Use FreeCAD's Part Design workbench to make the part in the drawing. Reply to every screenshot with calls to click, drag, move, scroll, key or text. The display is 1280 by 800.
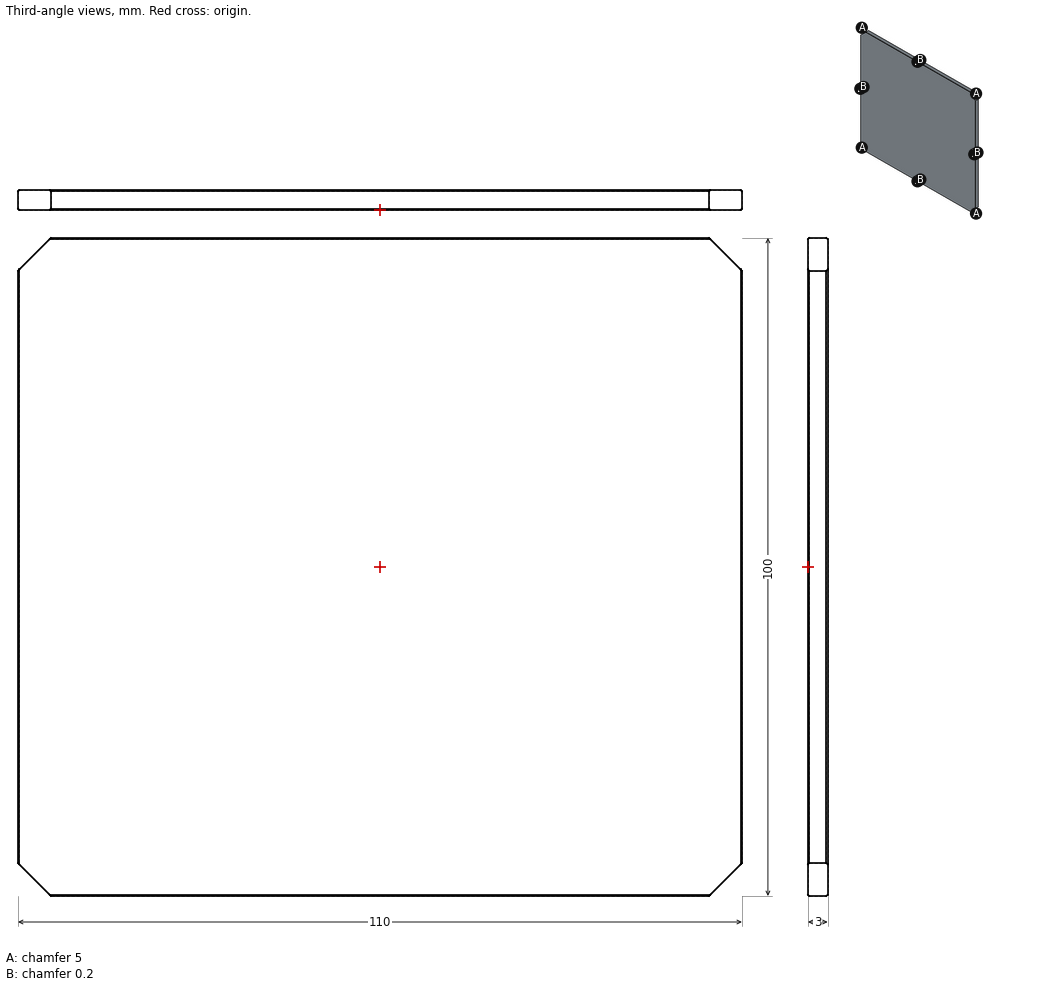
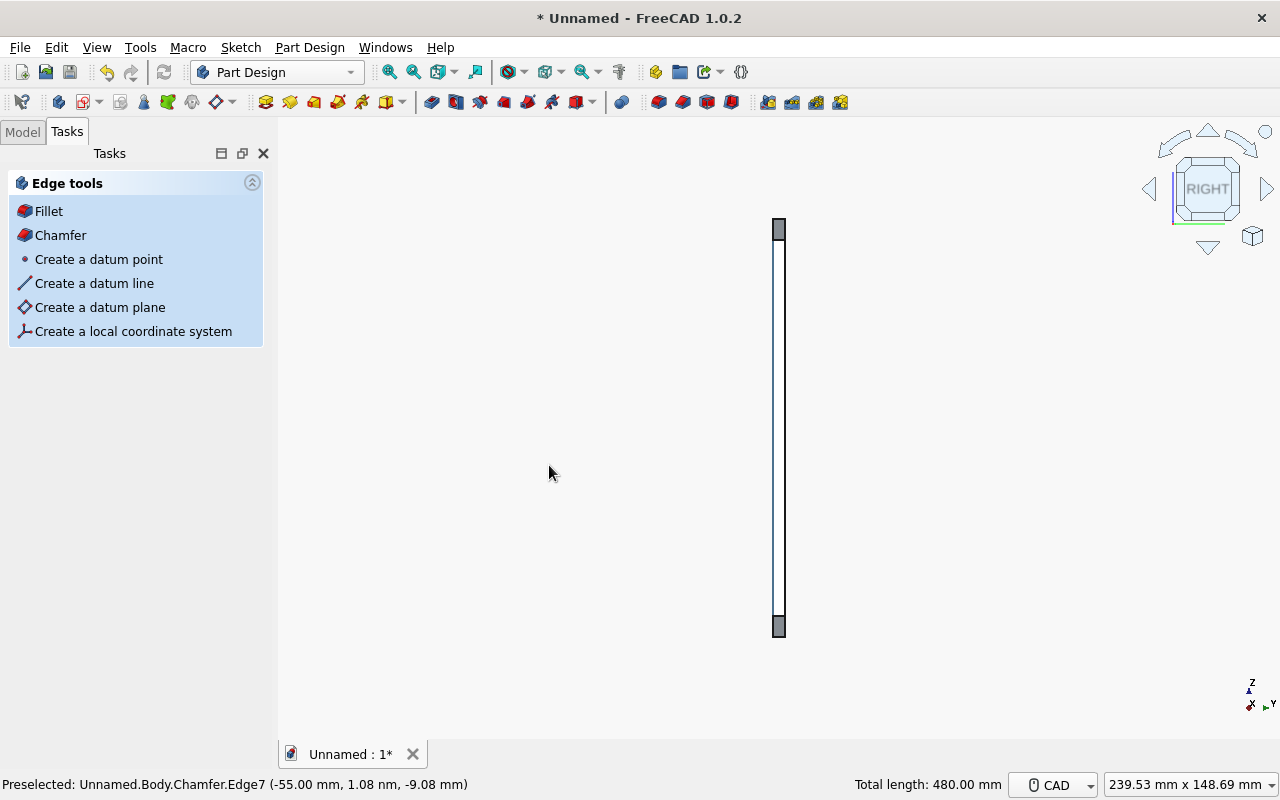
click(785, 427, ctrl)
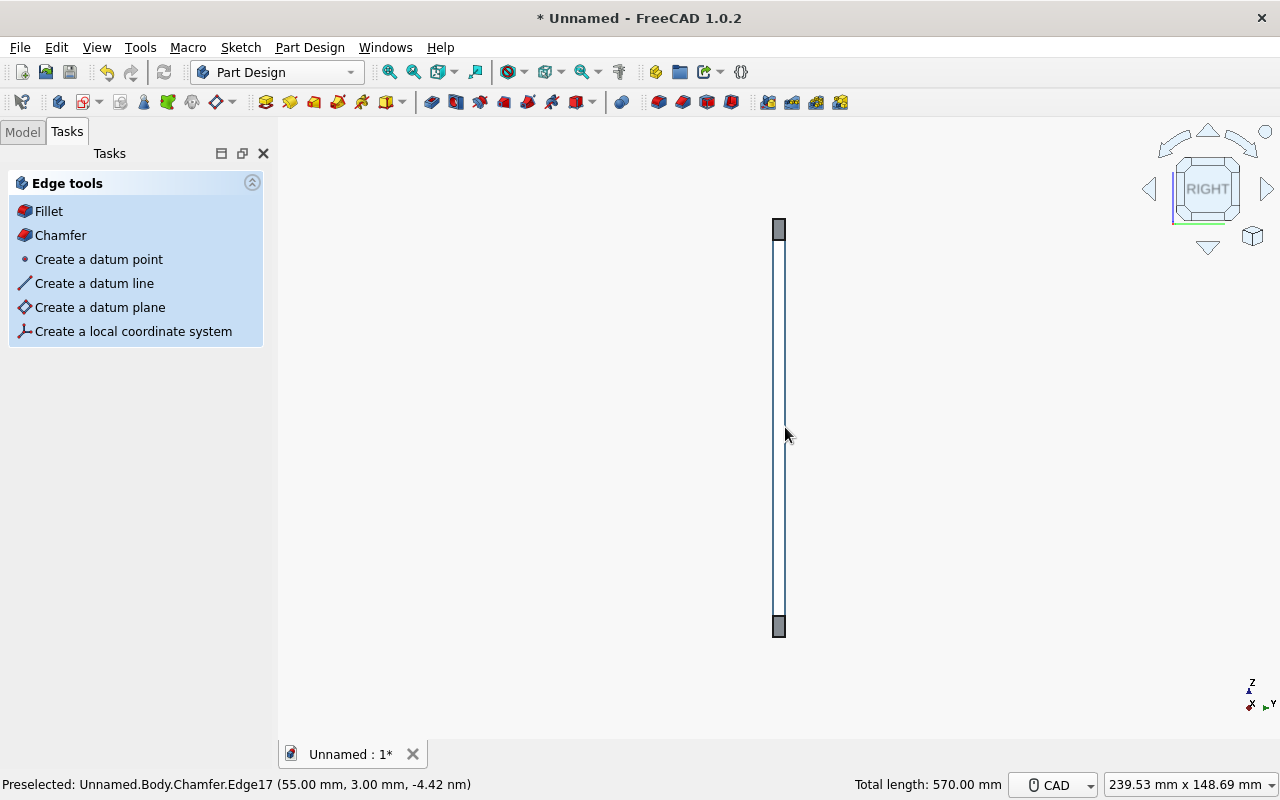
key(5)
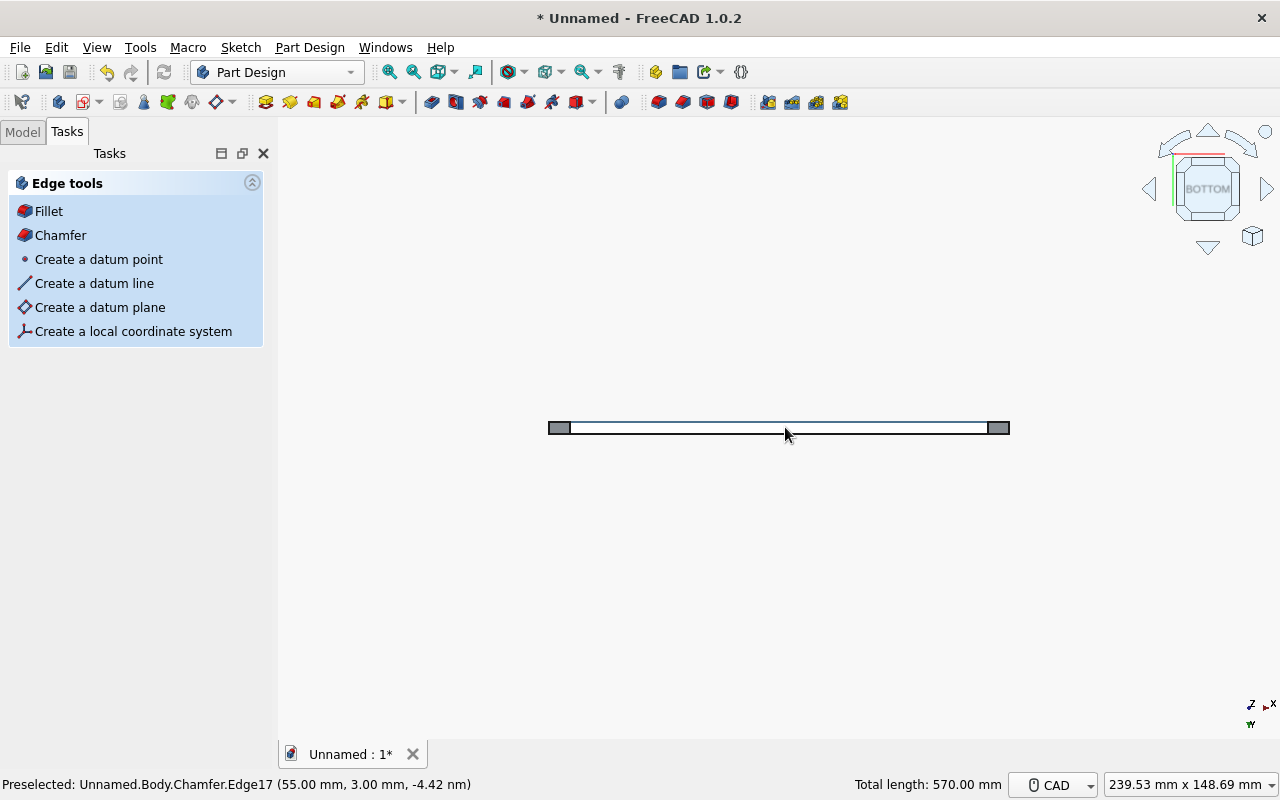
key(4)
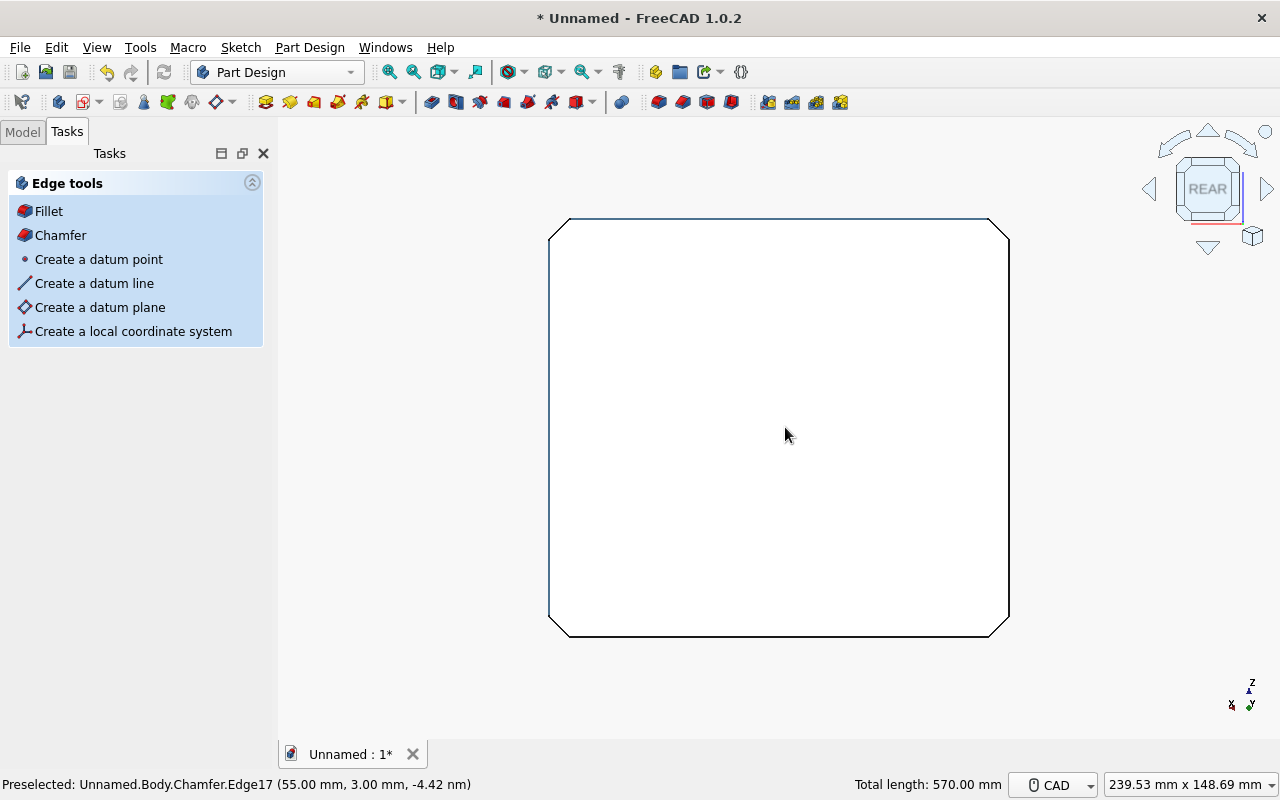
click(1009, 427, ctrl)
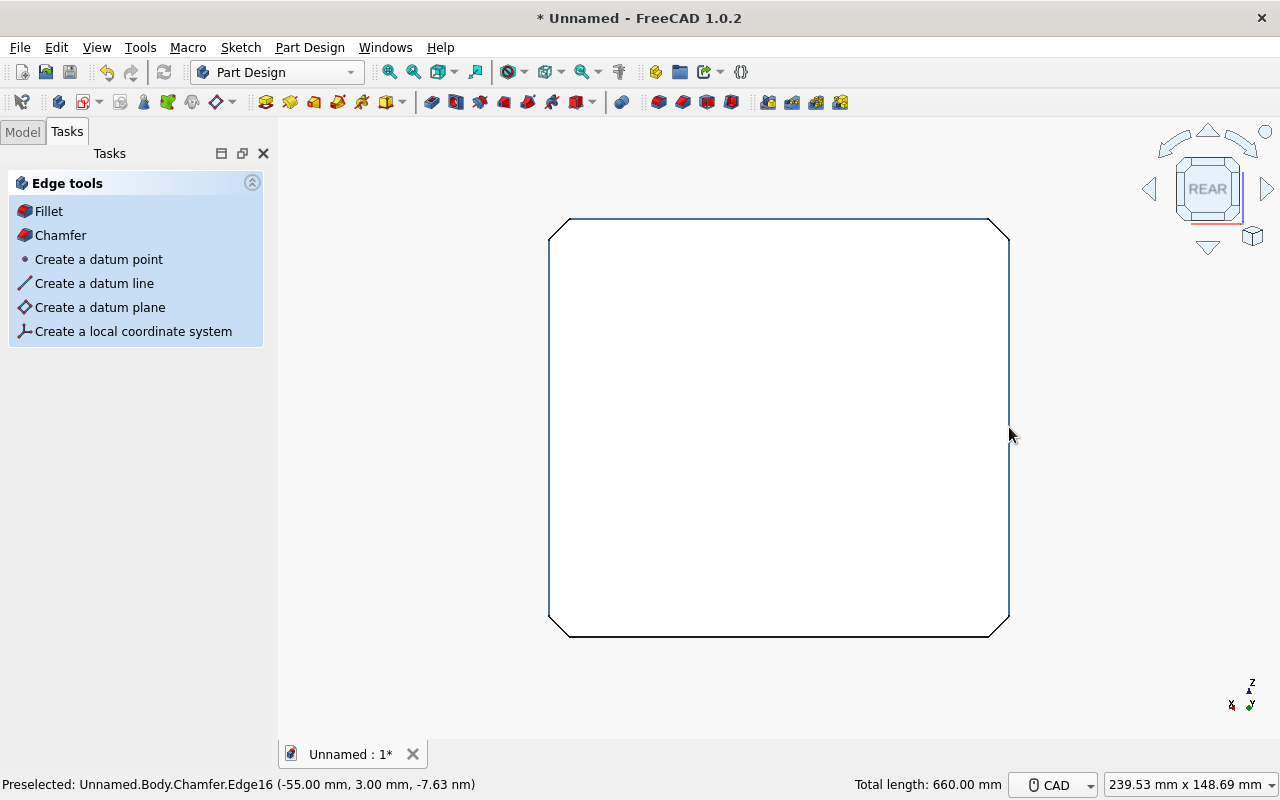
click(779, 636, ctrl)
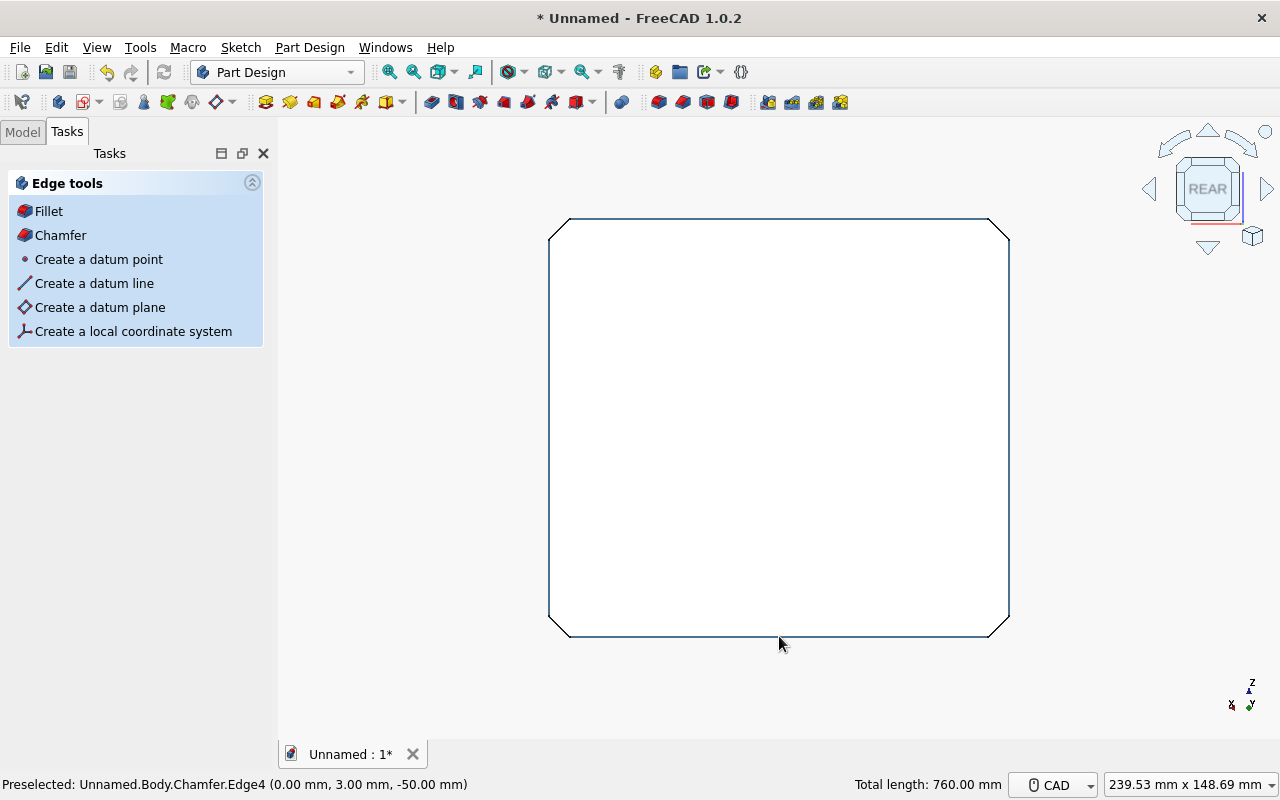
click(684, 102)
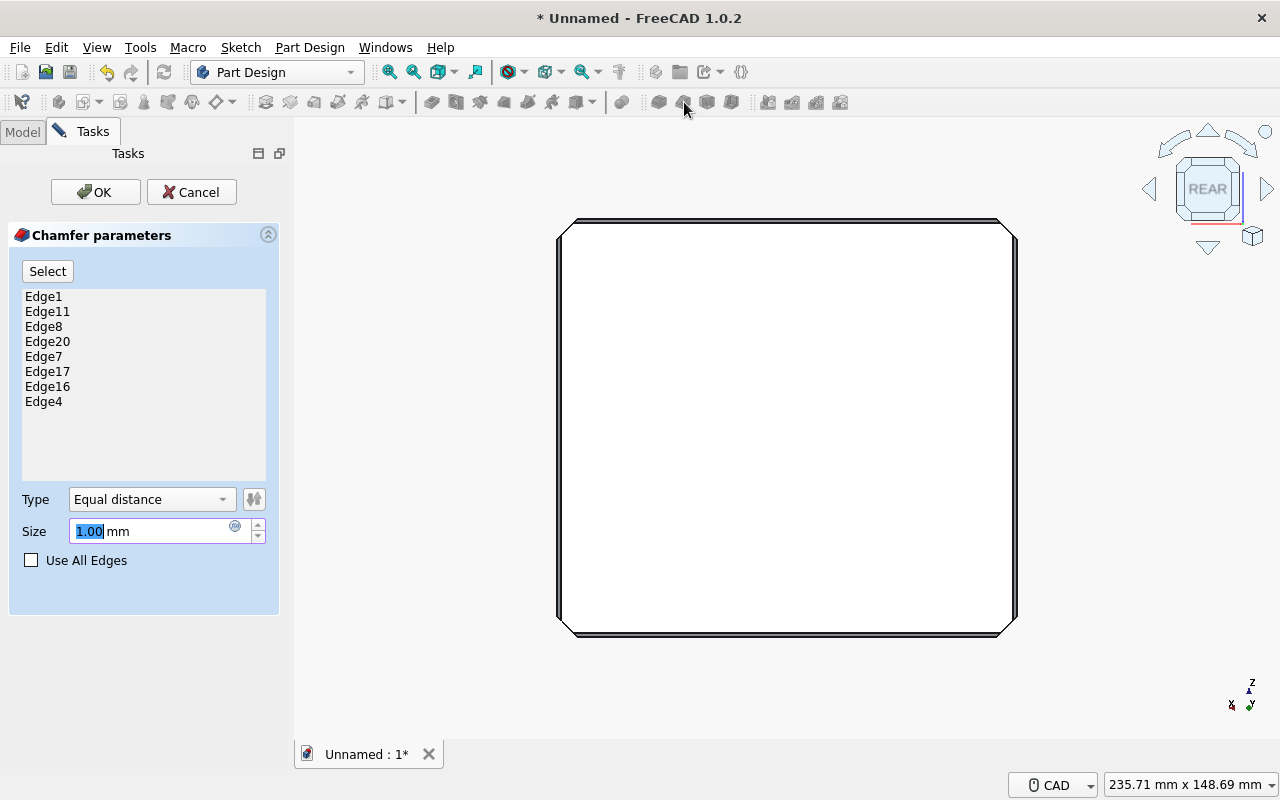
text(0.2)
key(Tab)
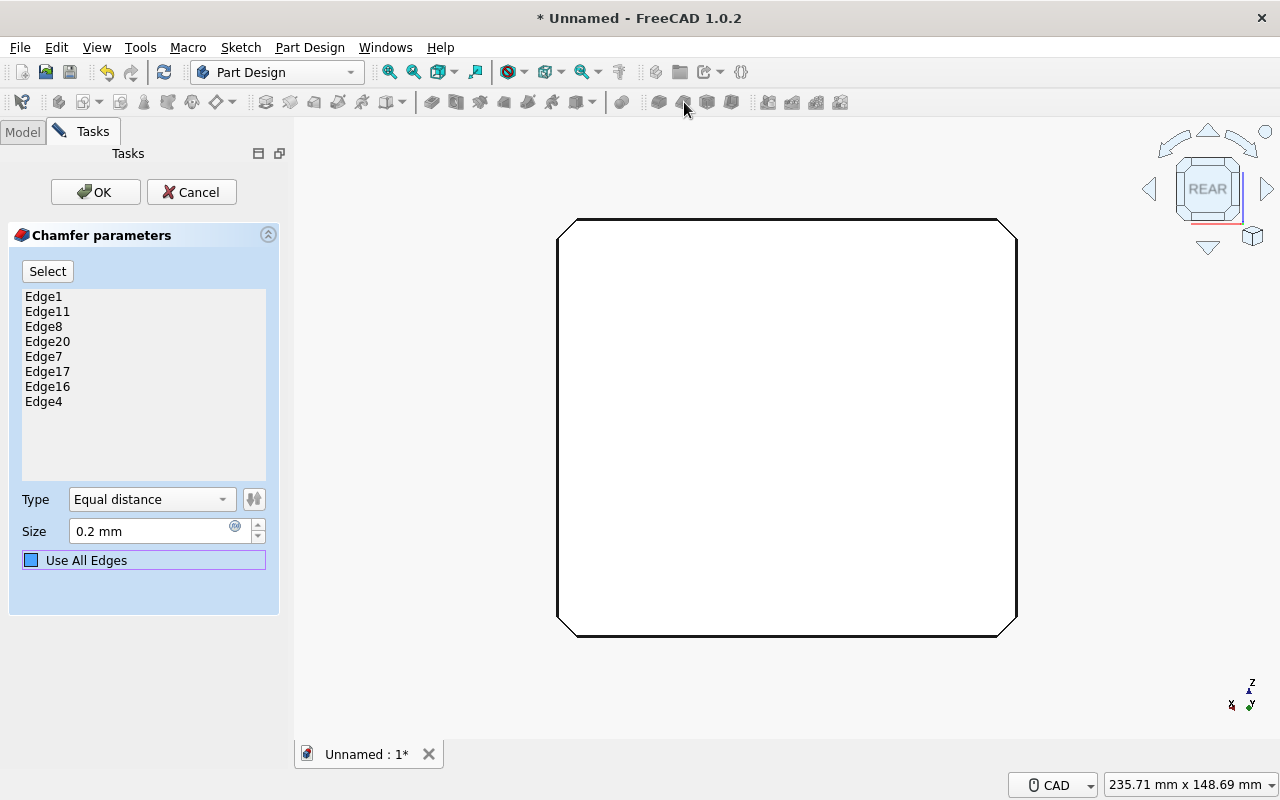
click(96, 192)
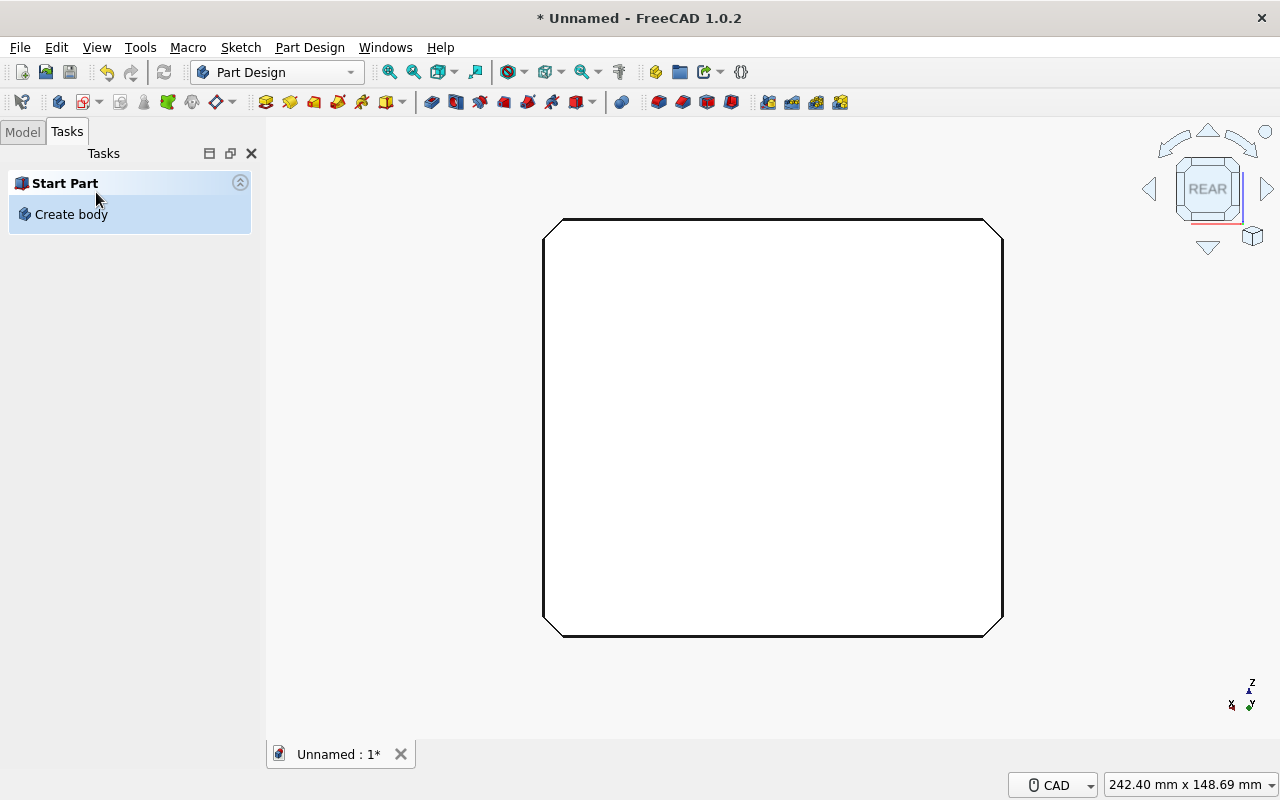
key(0)